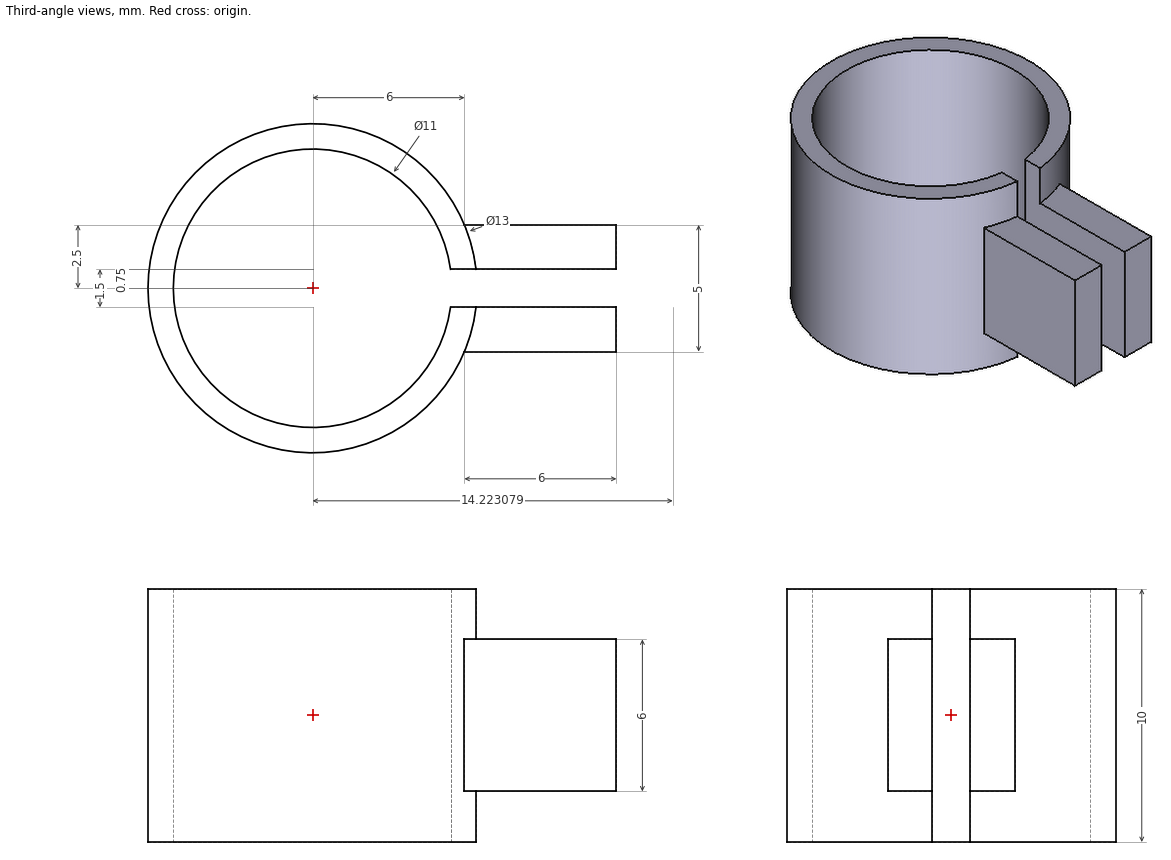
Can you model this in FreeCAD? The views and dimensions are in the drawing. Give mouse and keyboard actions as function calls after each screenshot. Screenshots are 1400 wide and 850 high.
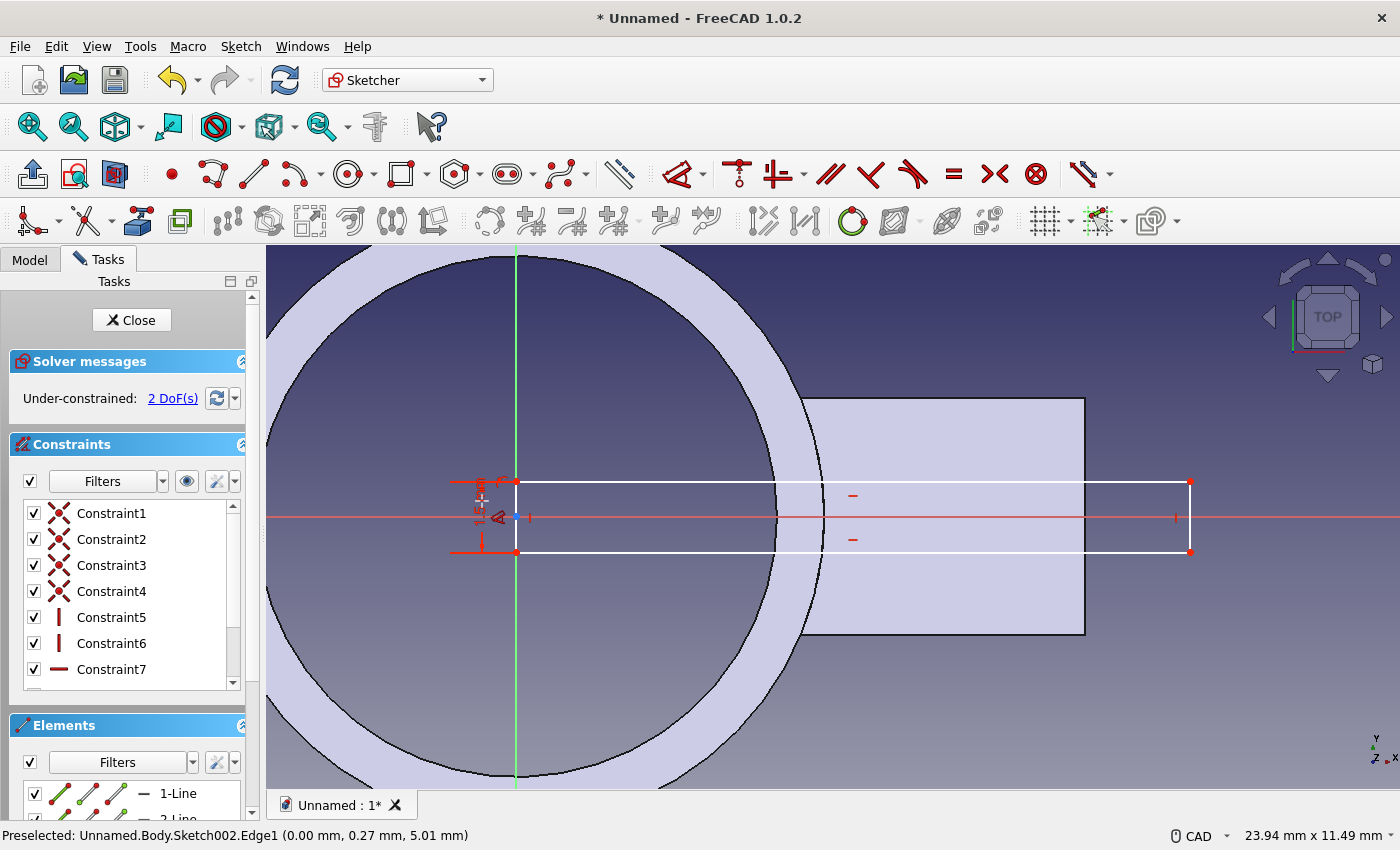
click(516, 482)
click(574, 499)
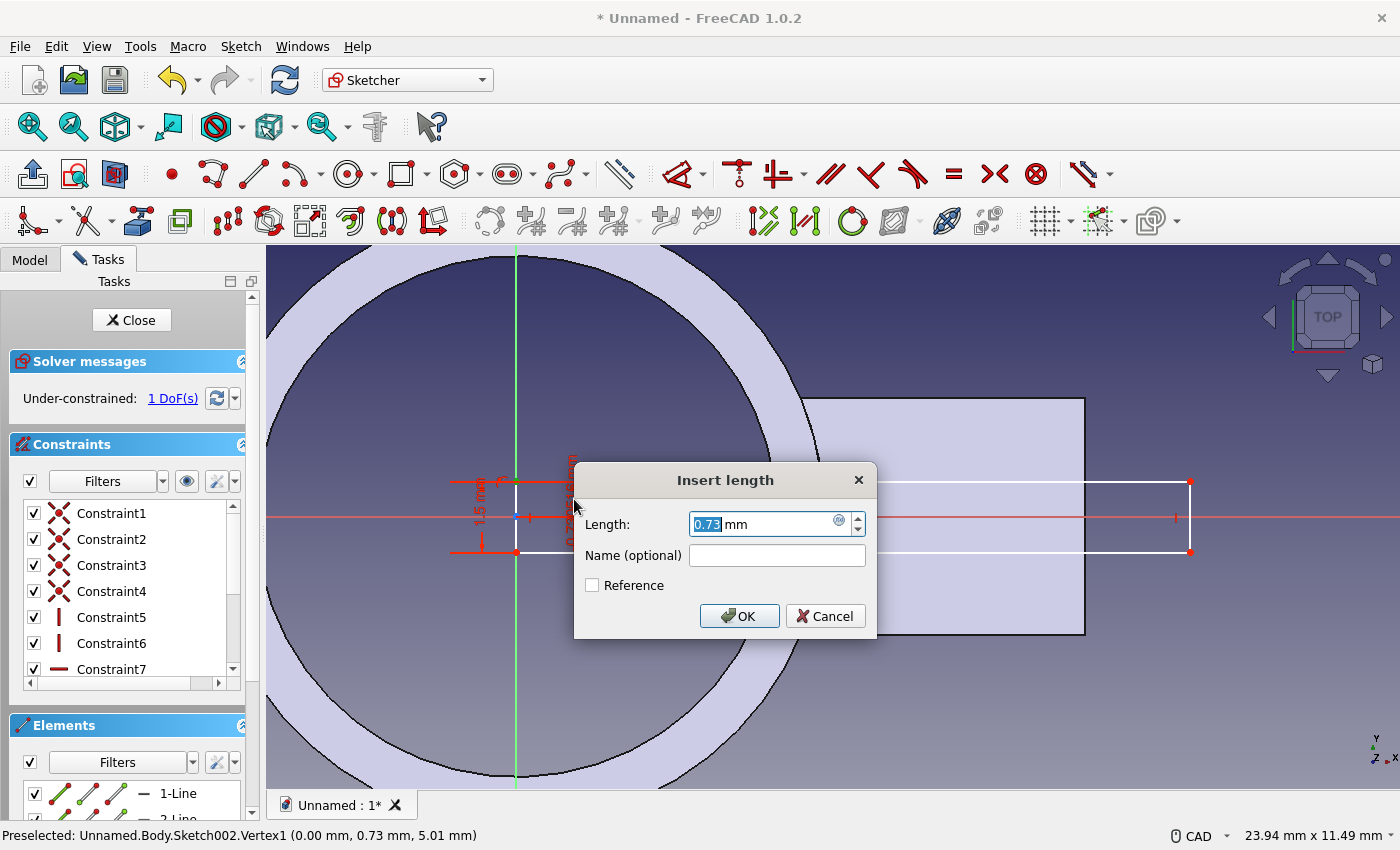
text(0.75)
key(Return)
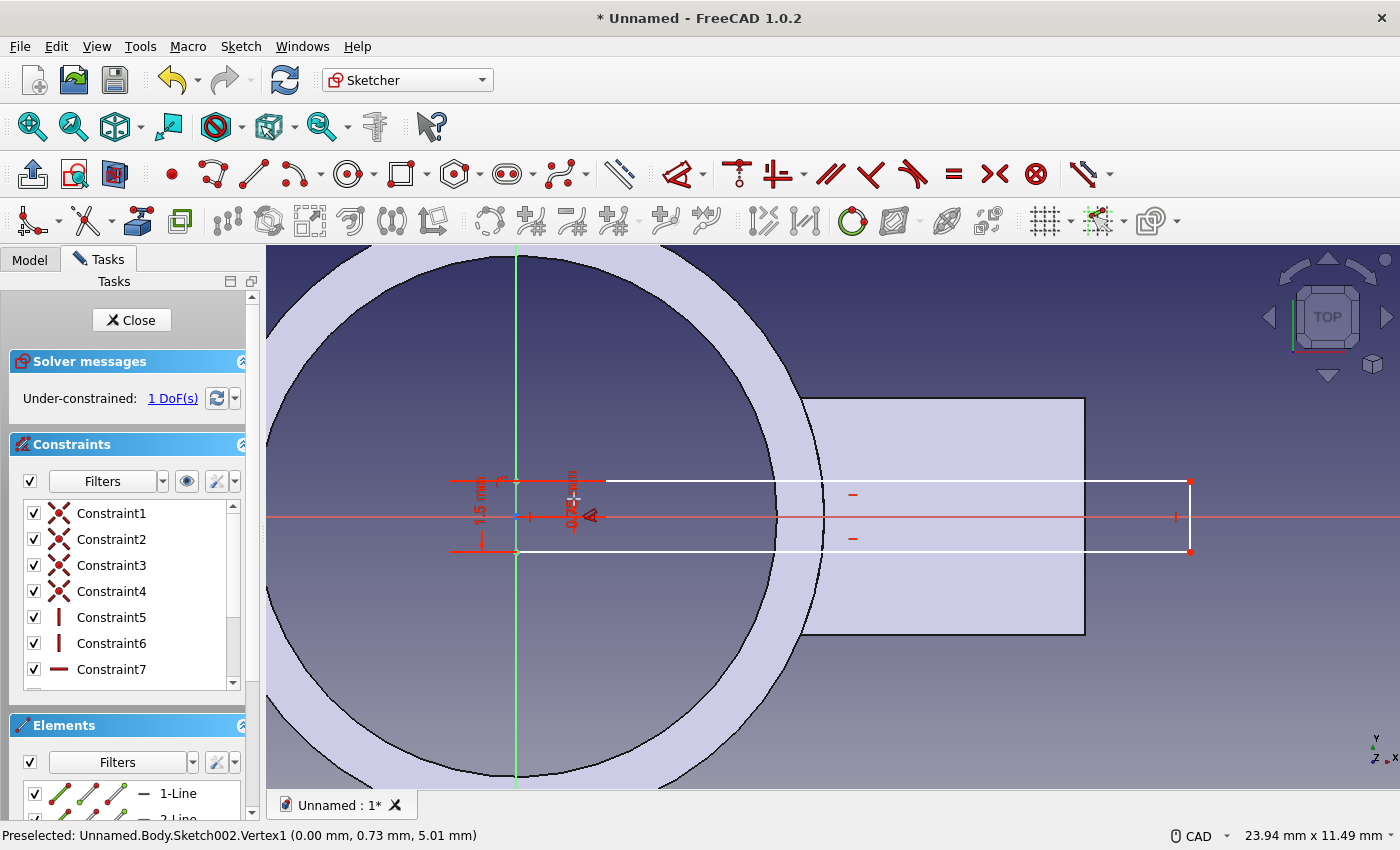
click(719, 552)
click(853, 586)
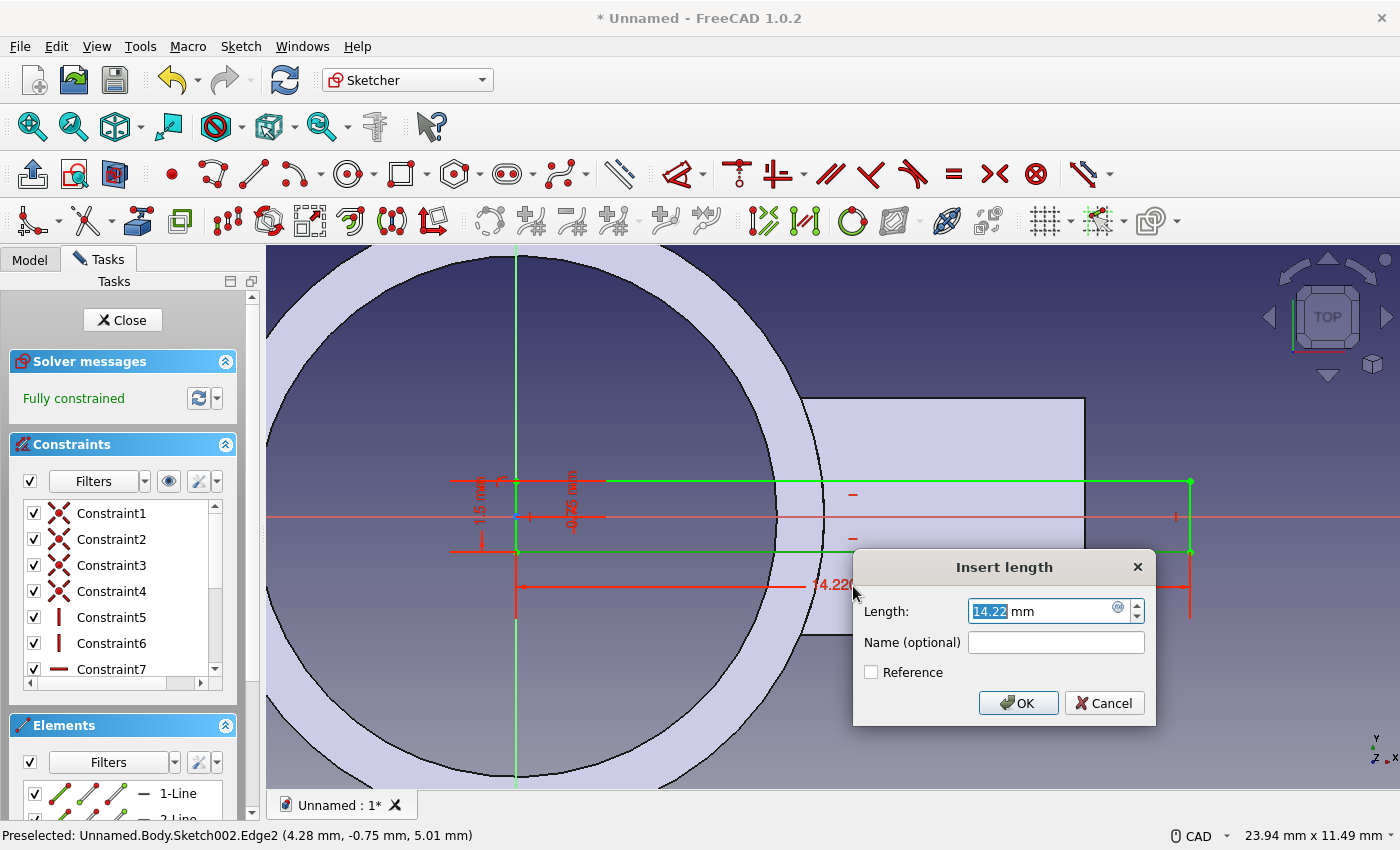
text(14.223079)
key(Return)
key(Escape)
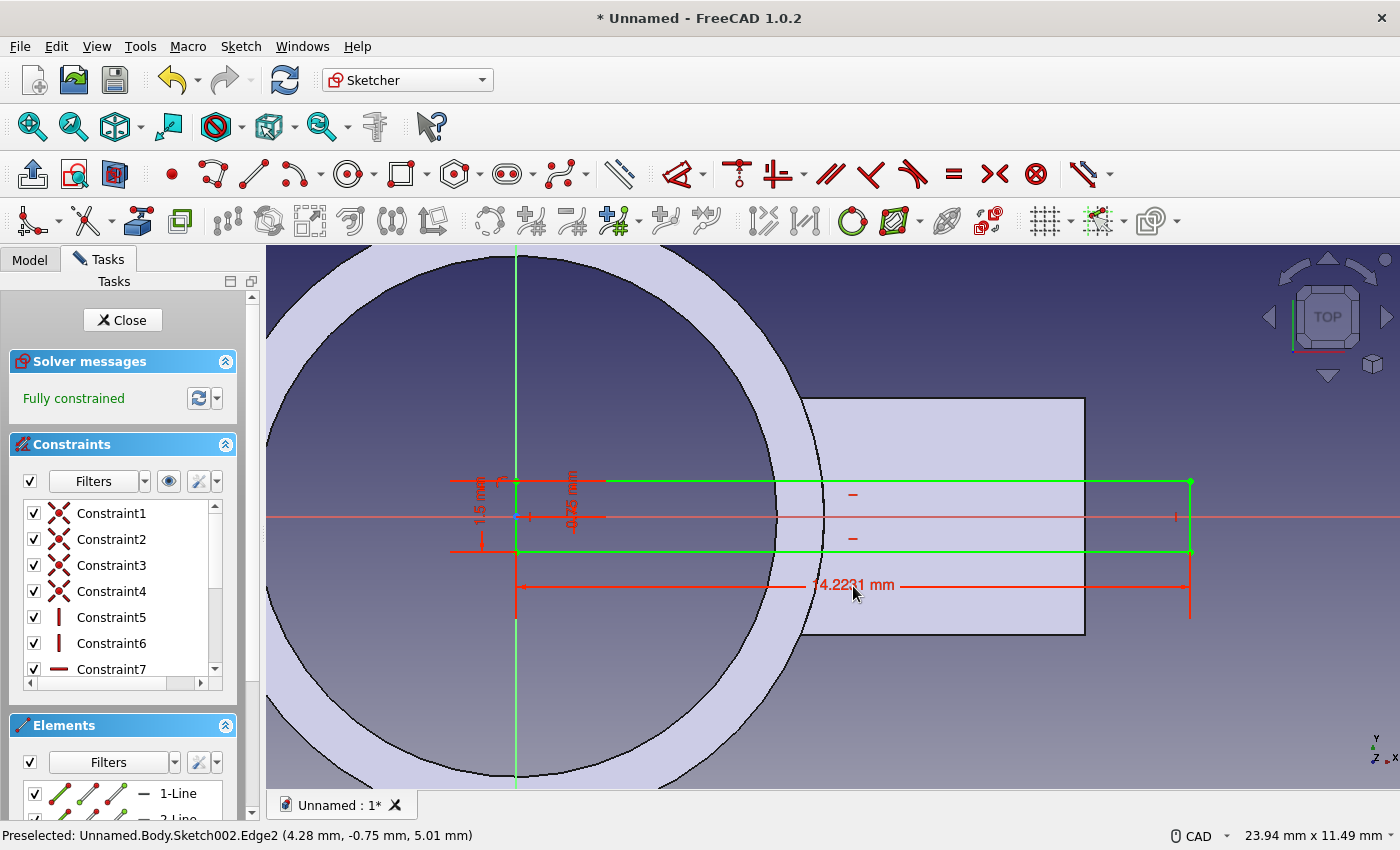
click(123, 320)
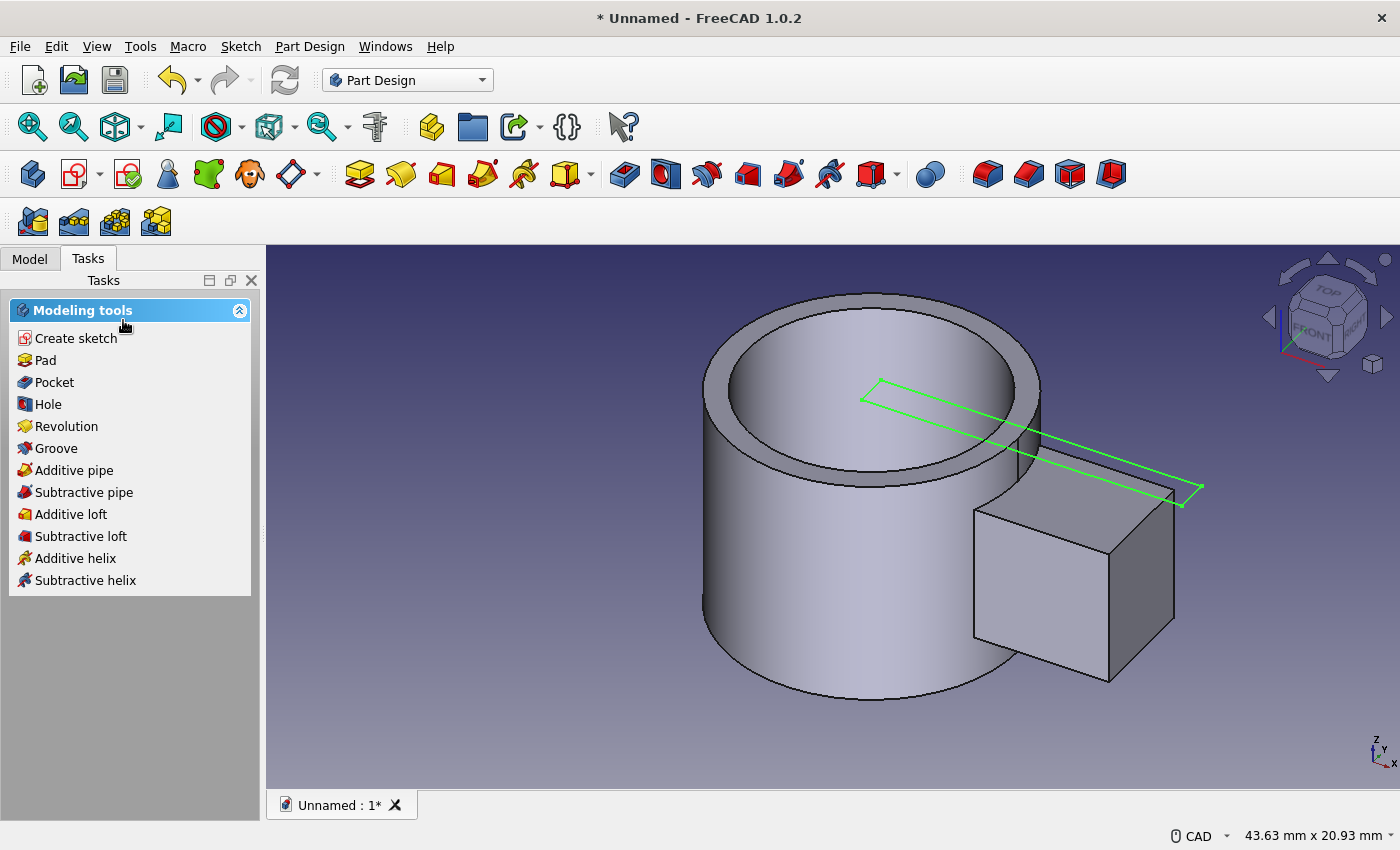
click(625, 174)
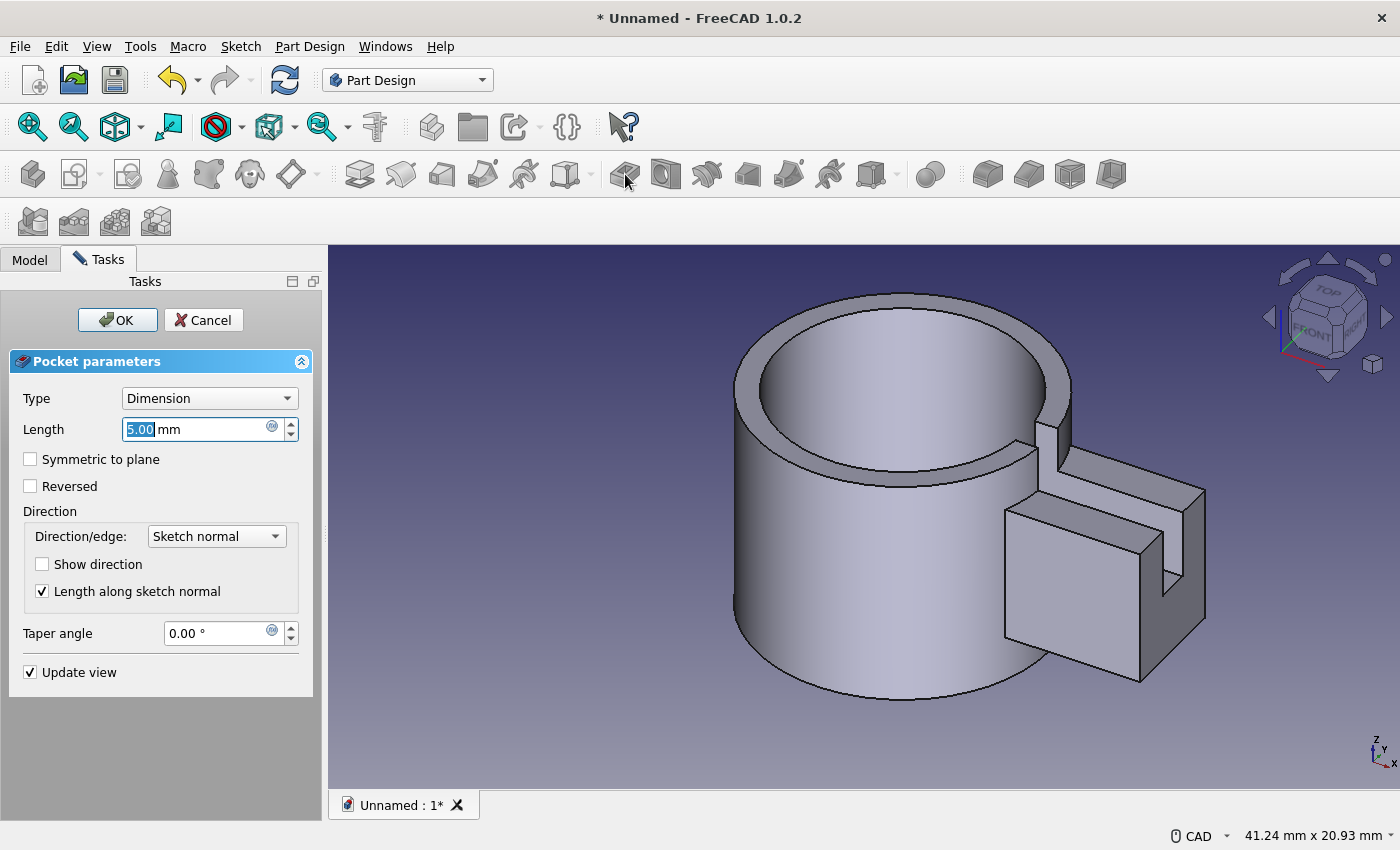
click(210, 398)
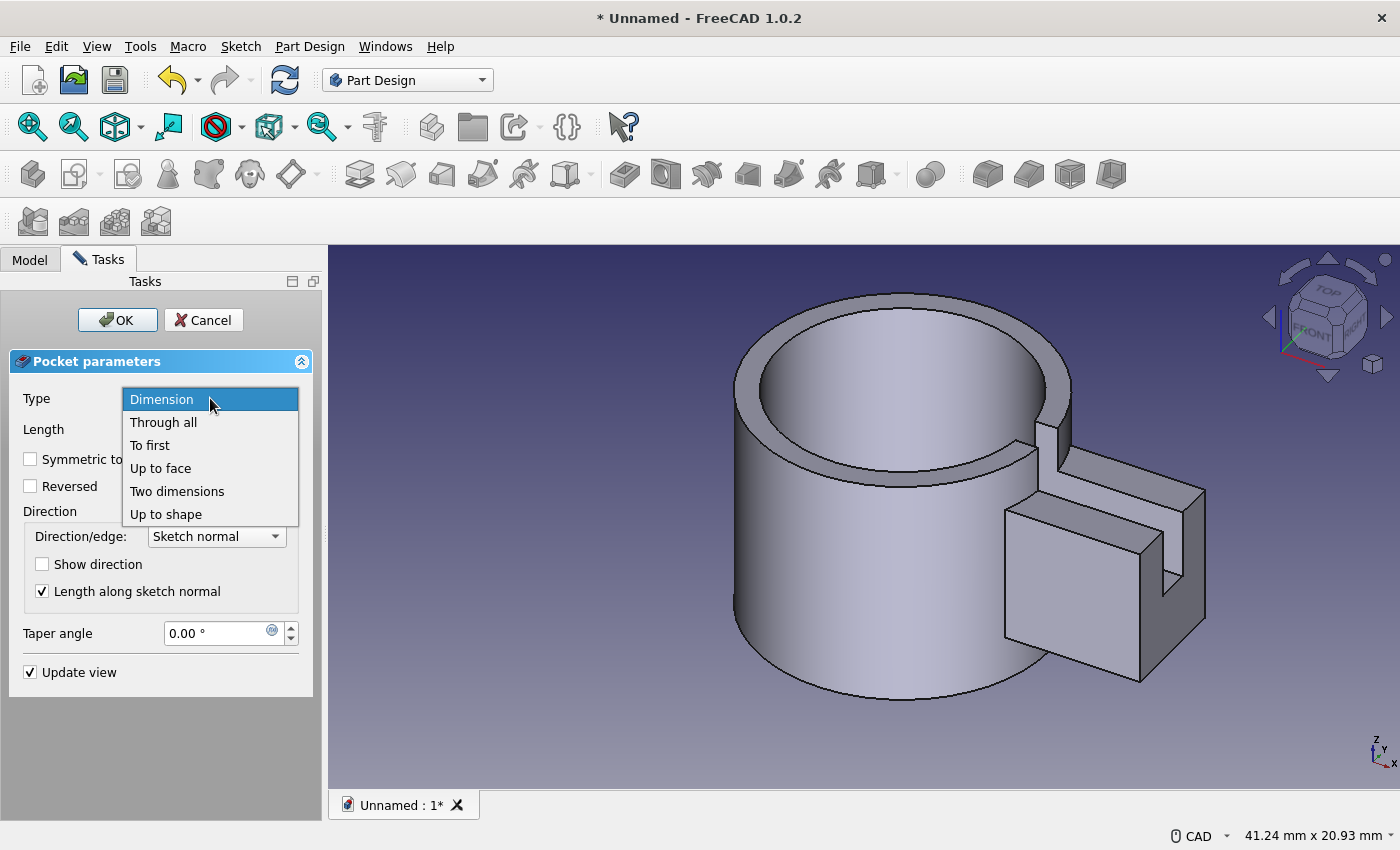
click(208, 422)